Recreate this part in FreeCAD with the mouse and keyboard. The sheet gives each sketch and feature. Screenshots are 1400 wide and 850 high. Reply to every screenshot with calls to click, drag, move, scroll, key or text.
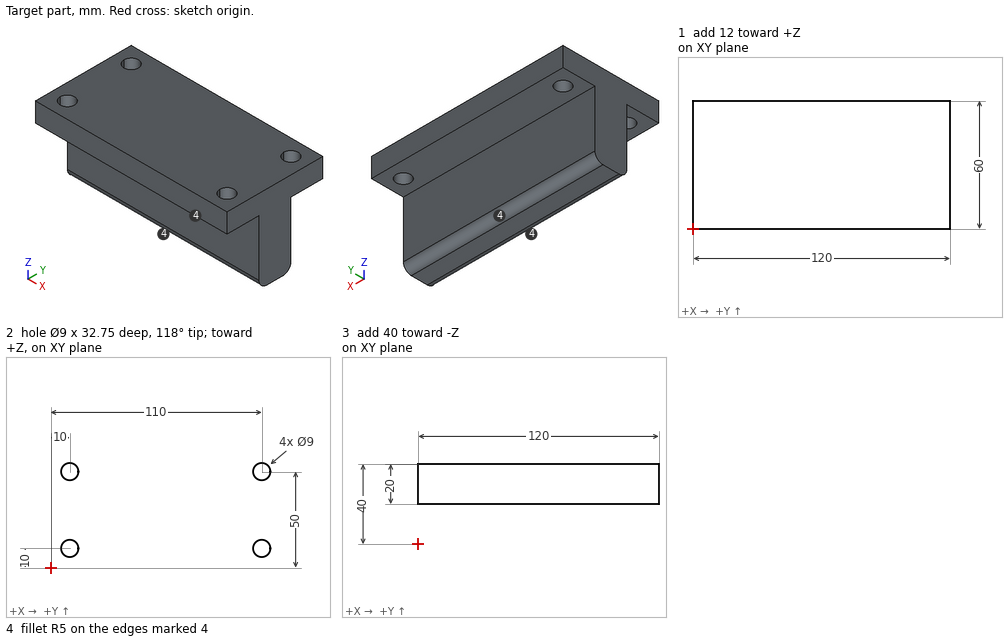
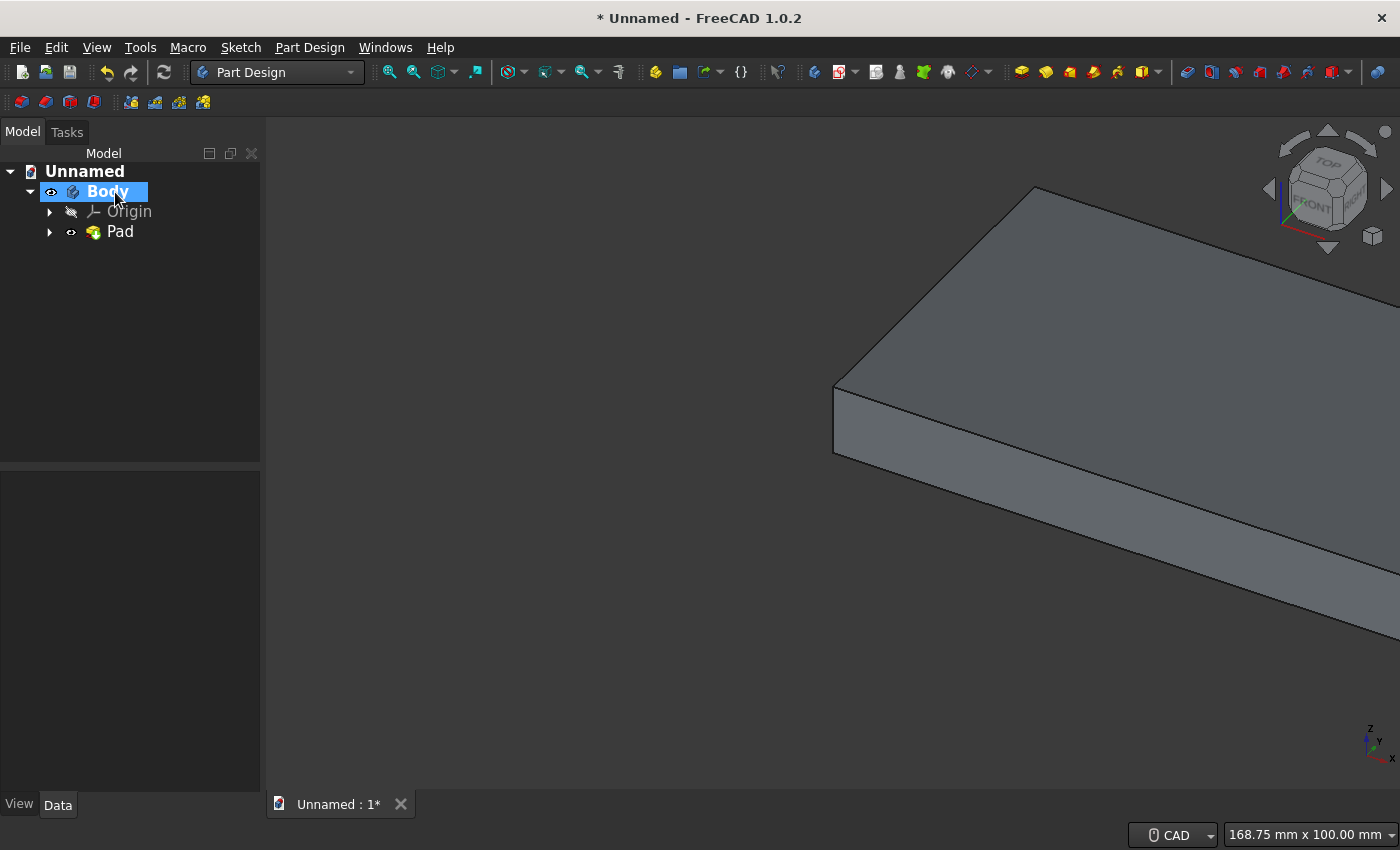
click(390, 72)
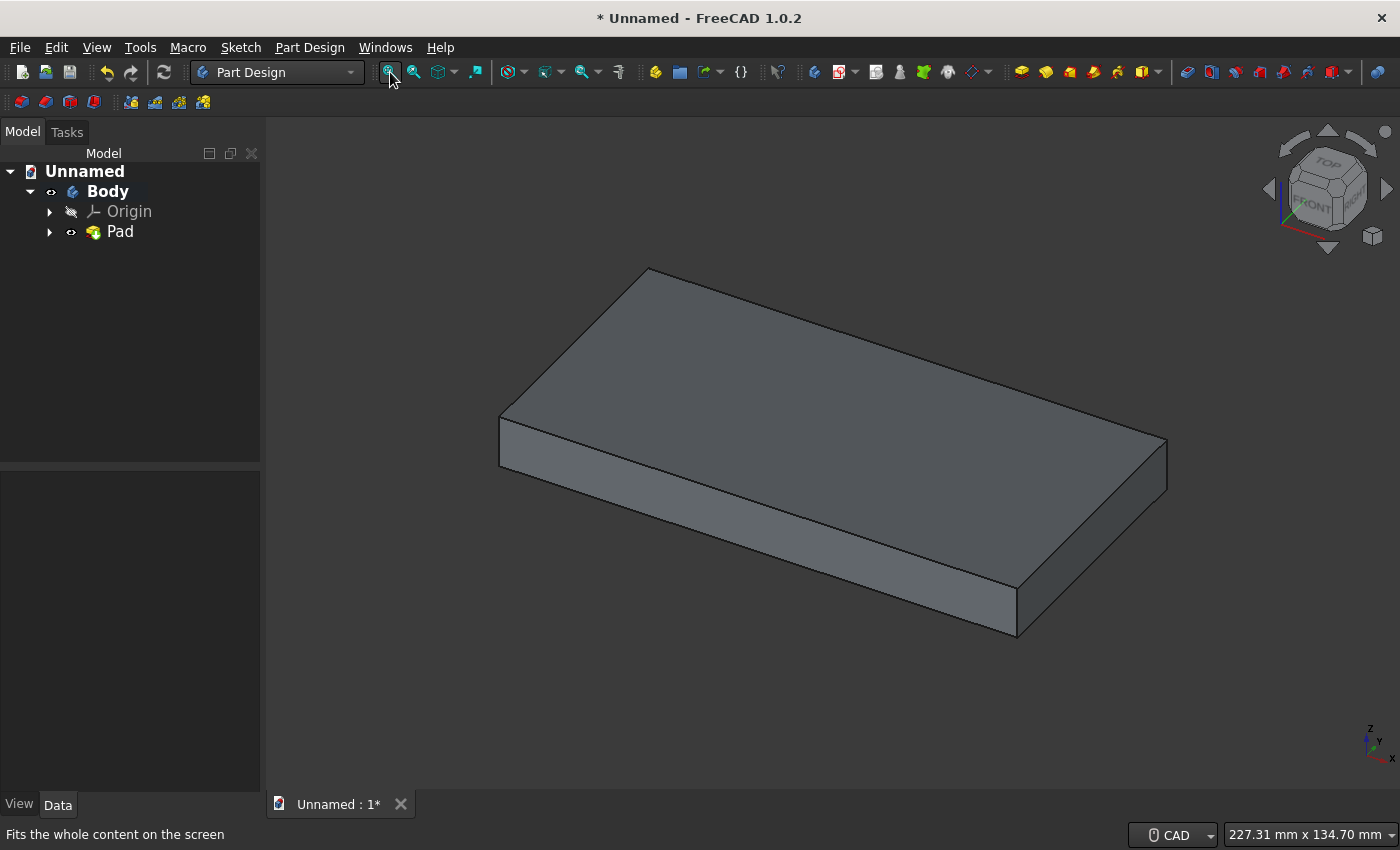
click(840, 72)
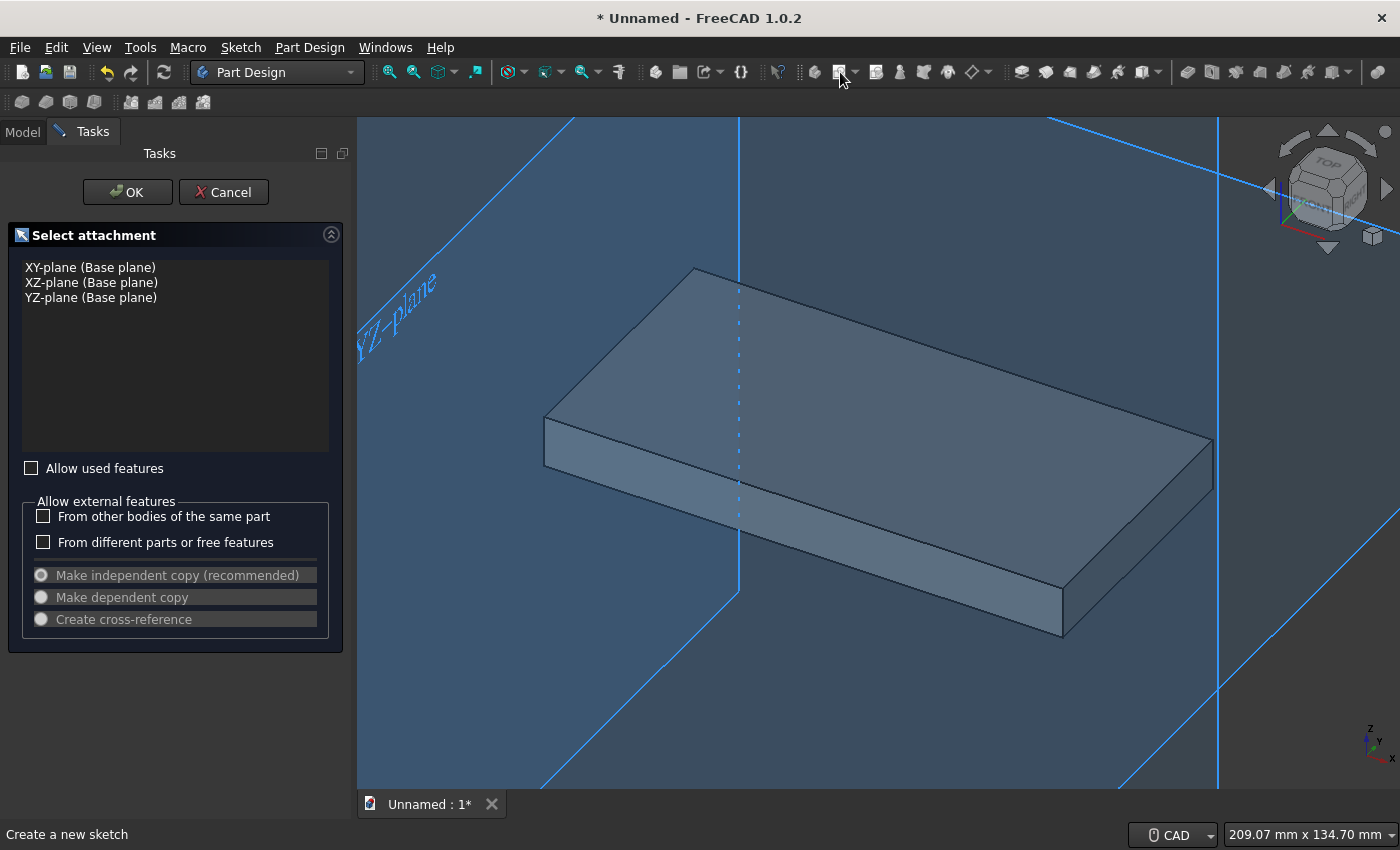
click(82, 268)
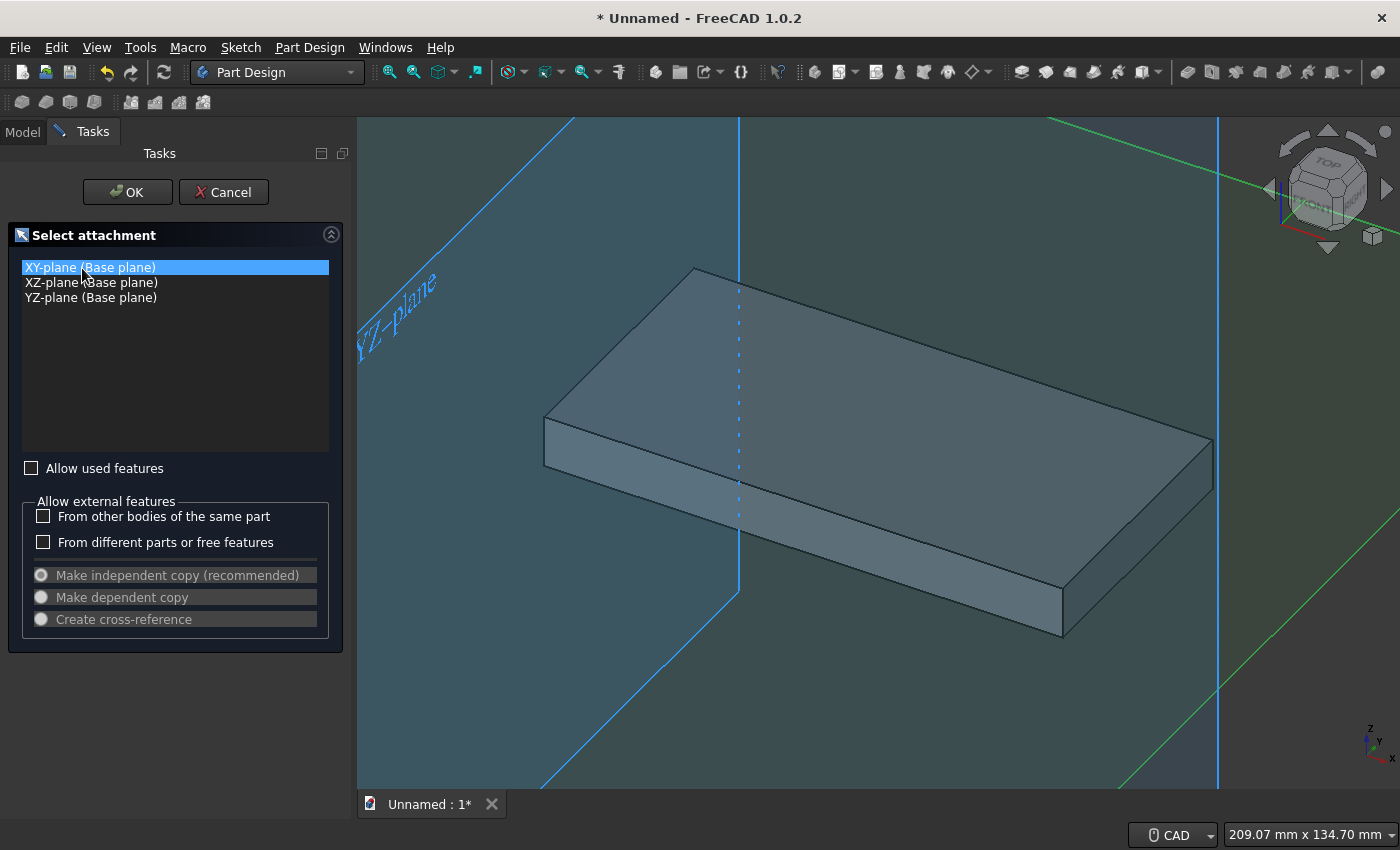
click(128, 192)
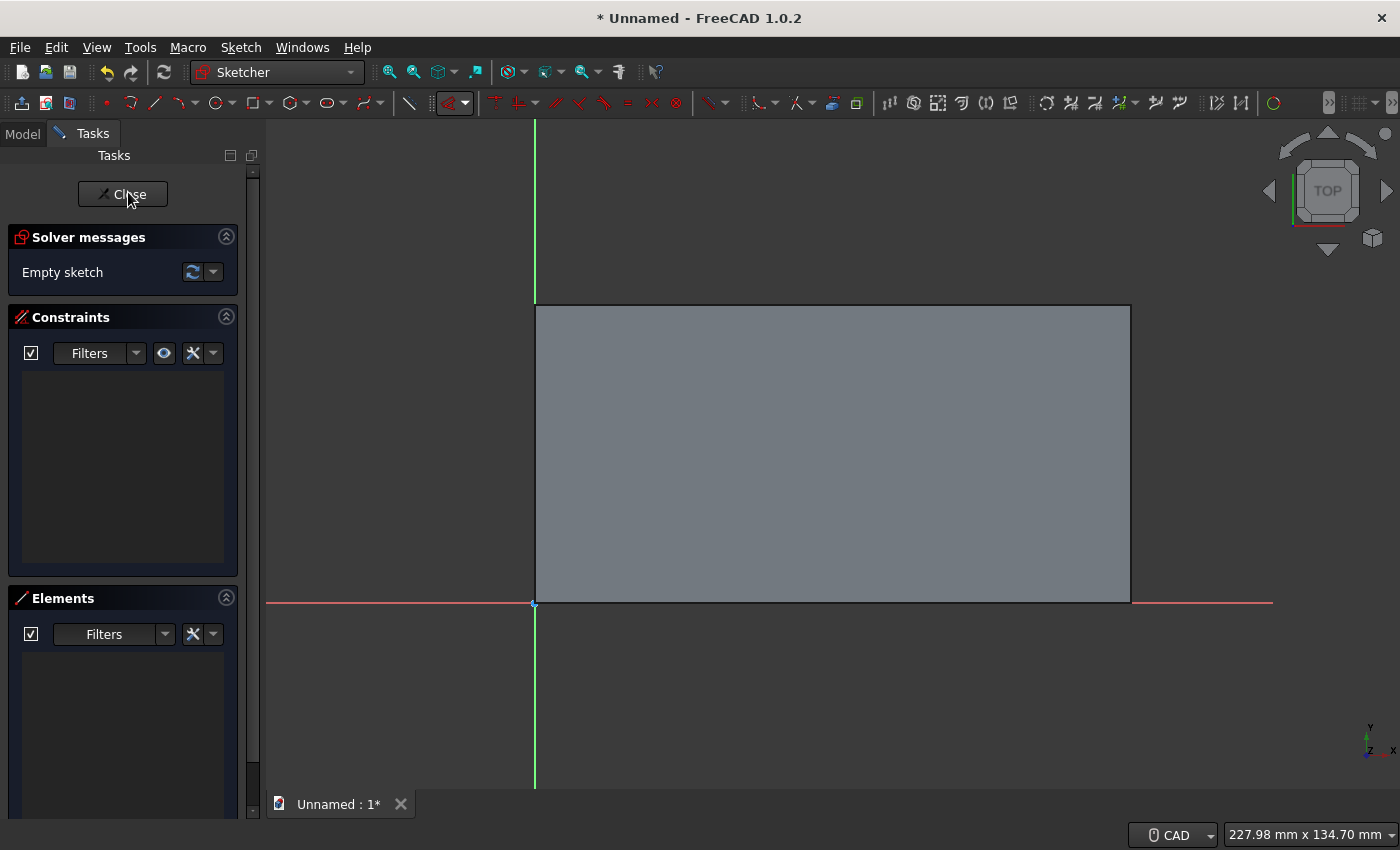
click(70, 104)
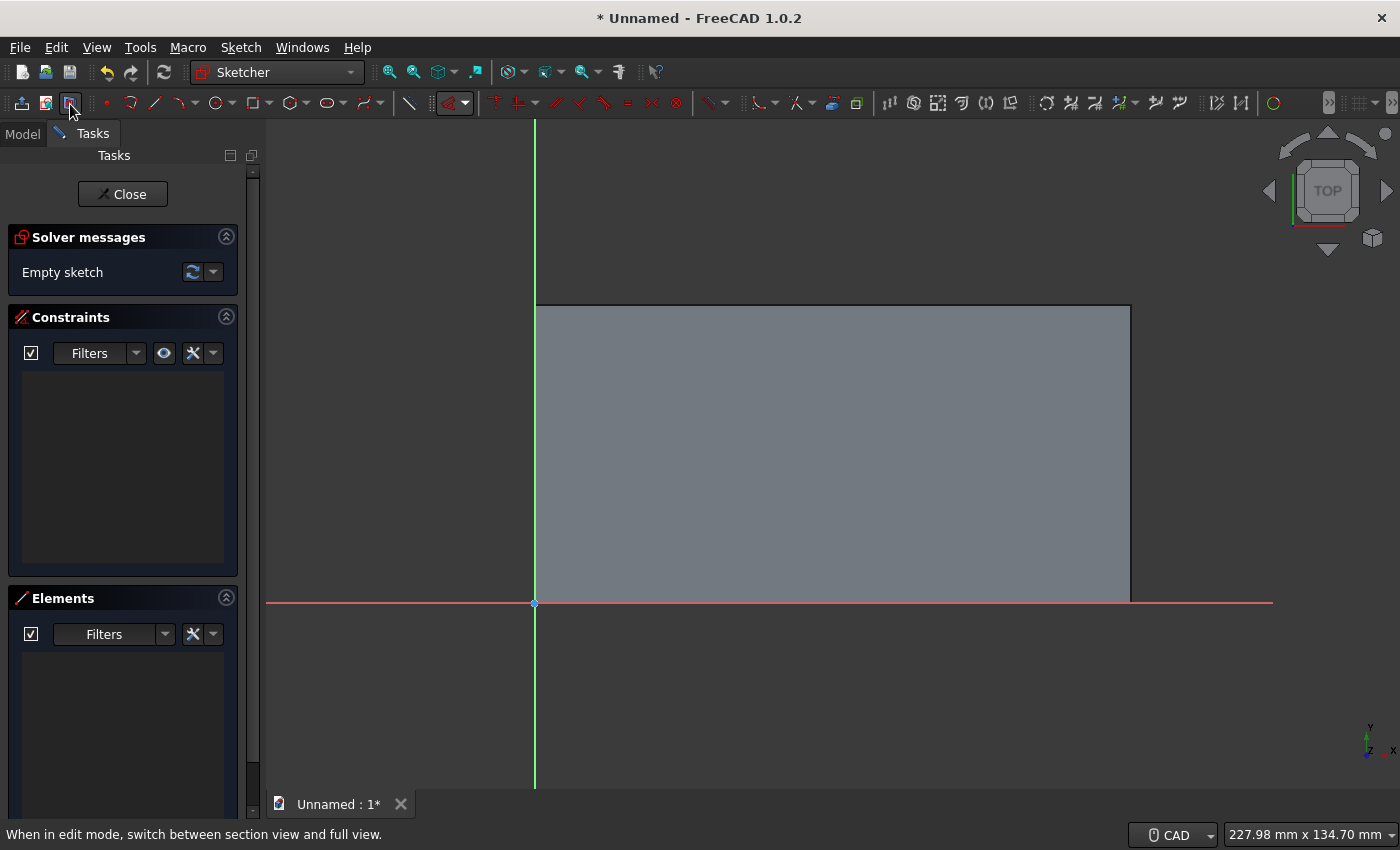
click(216, 104)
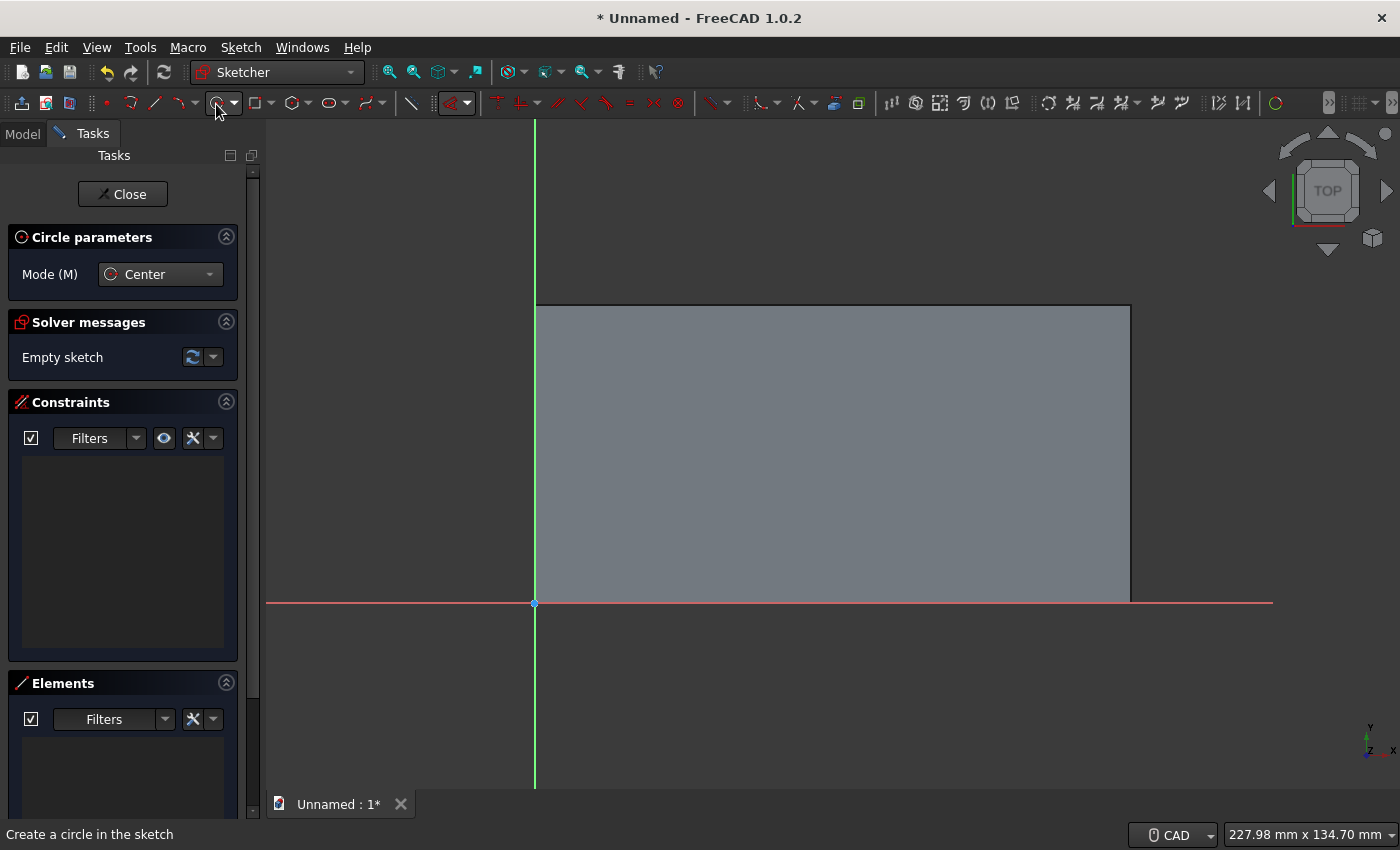
click(1082, 355)
click(1098, 339)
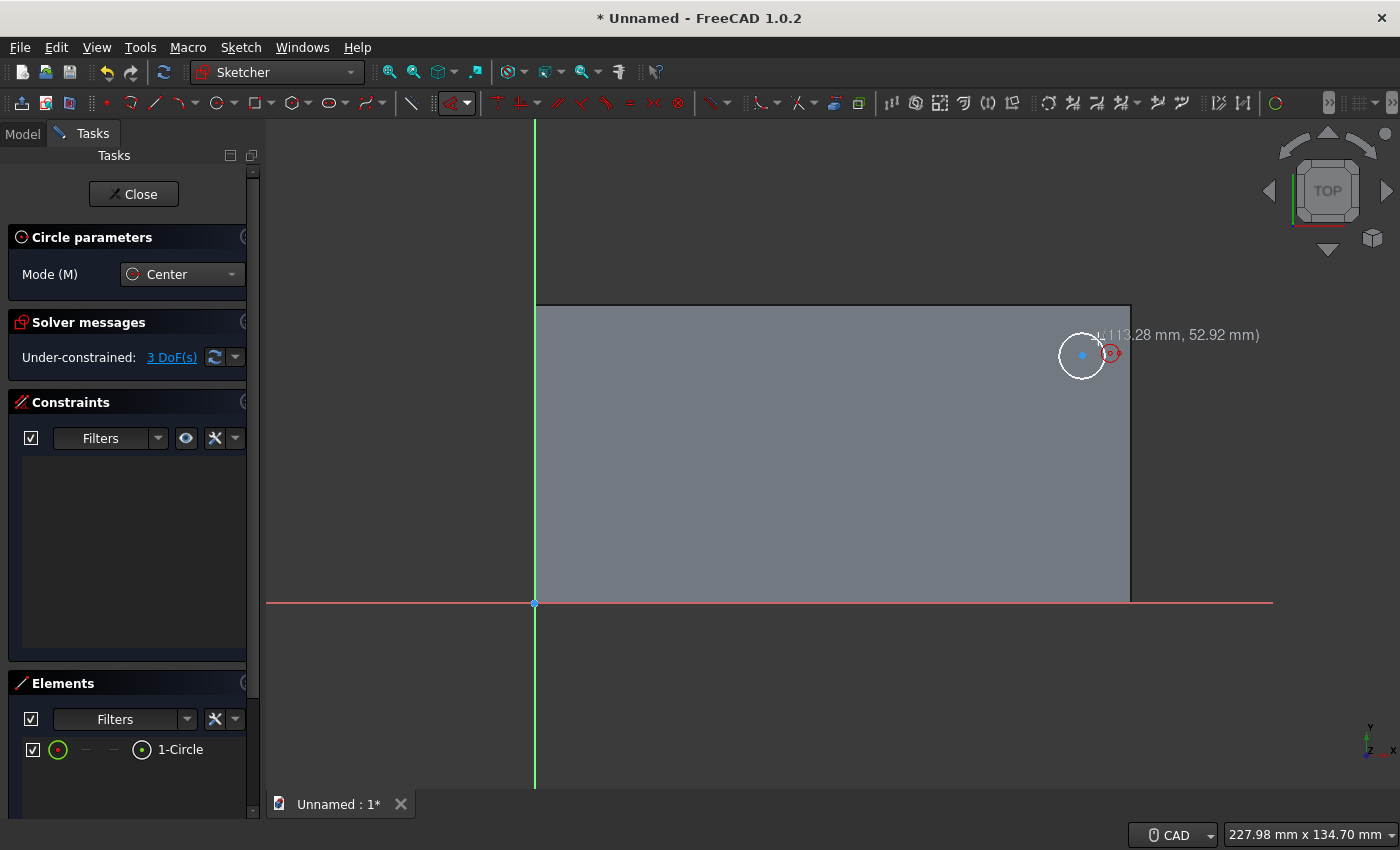
click(584, 355)
click(600, 339)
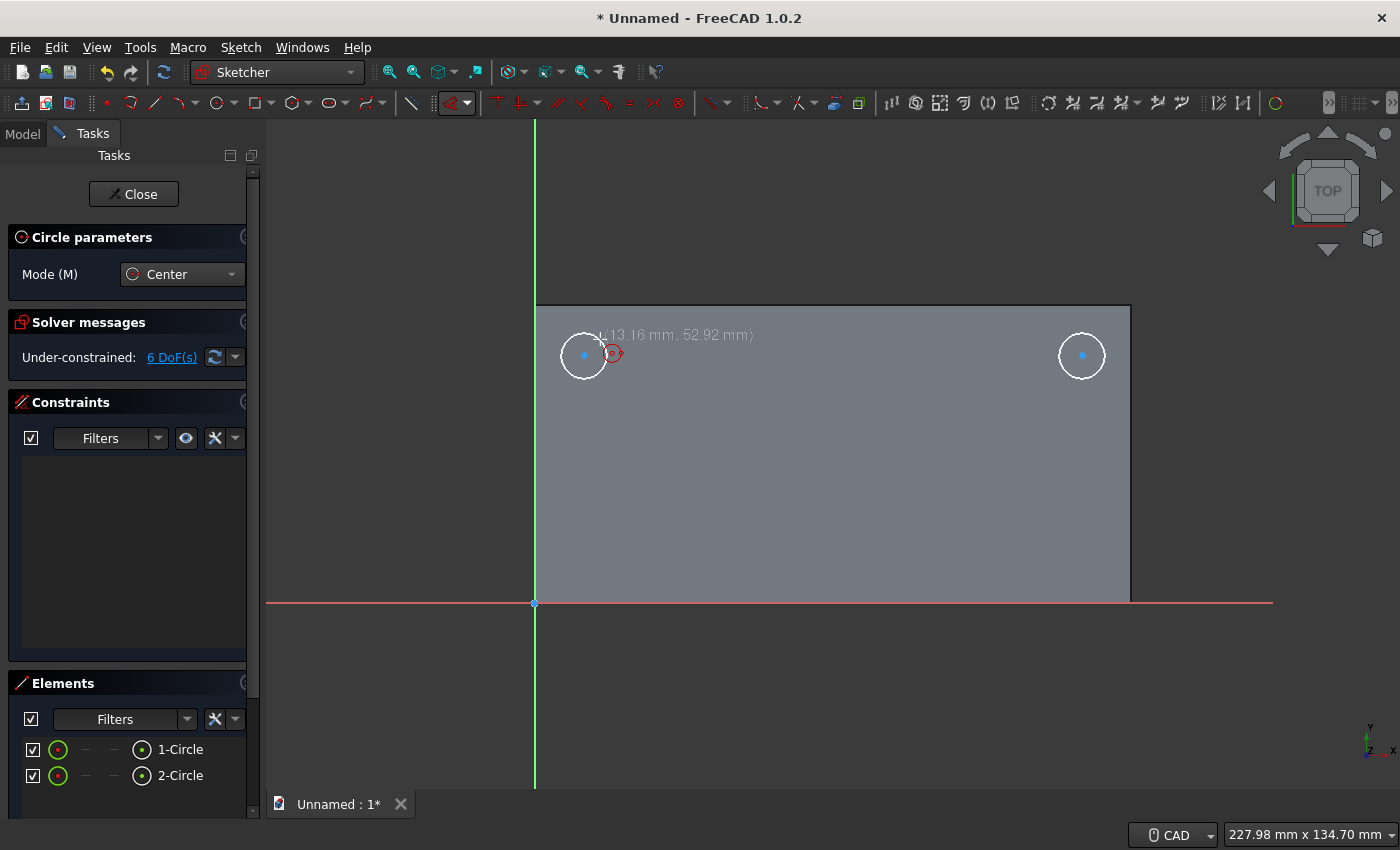
click(584, 553)
click(600, 538)